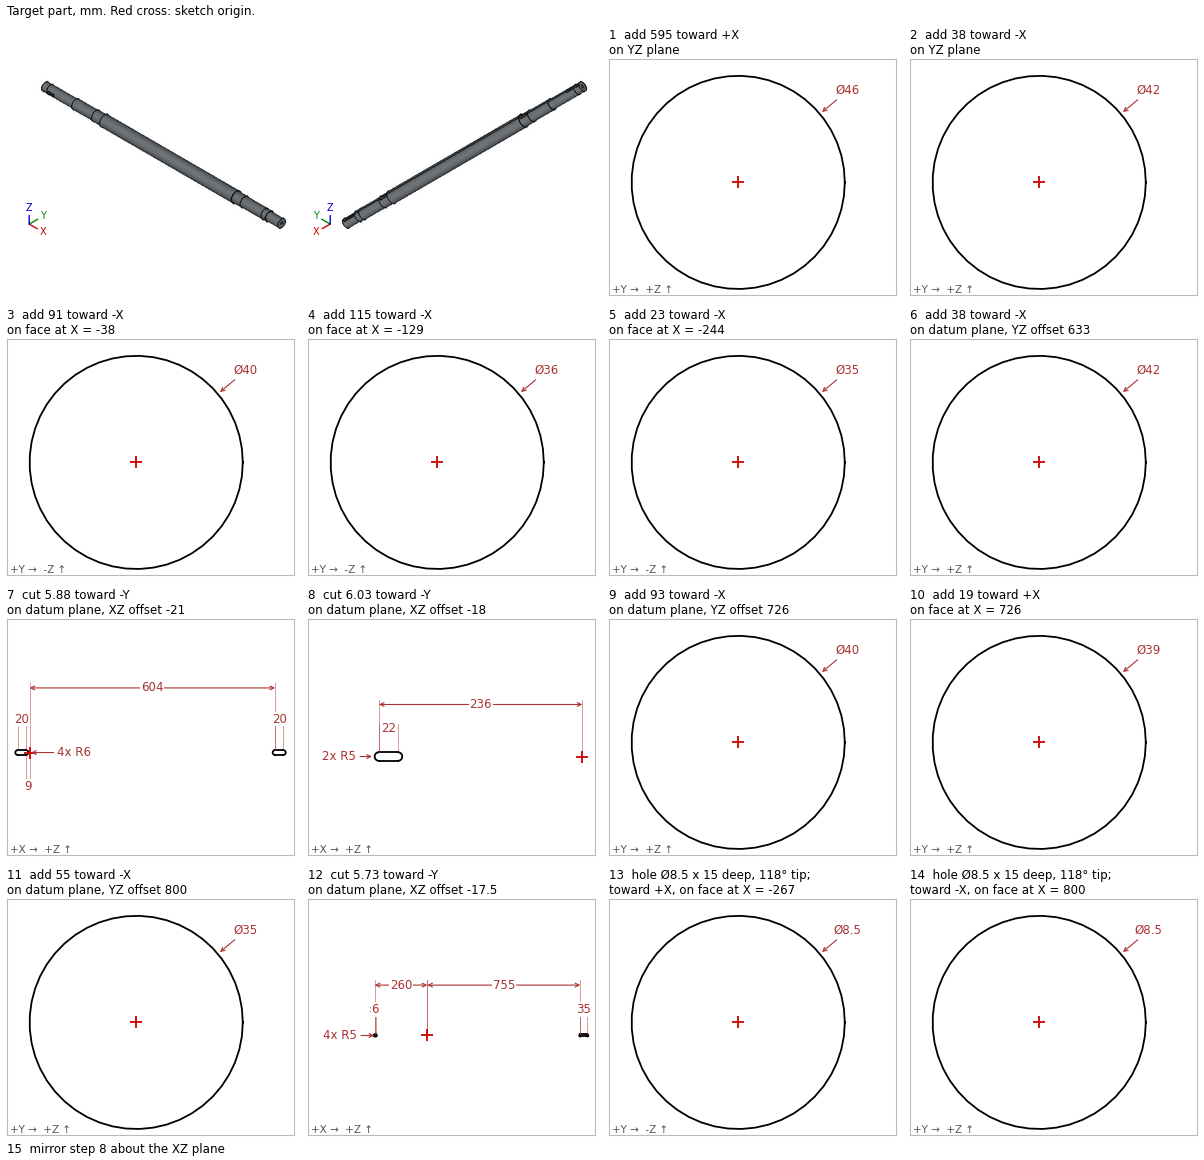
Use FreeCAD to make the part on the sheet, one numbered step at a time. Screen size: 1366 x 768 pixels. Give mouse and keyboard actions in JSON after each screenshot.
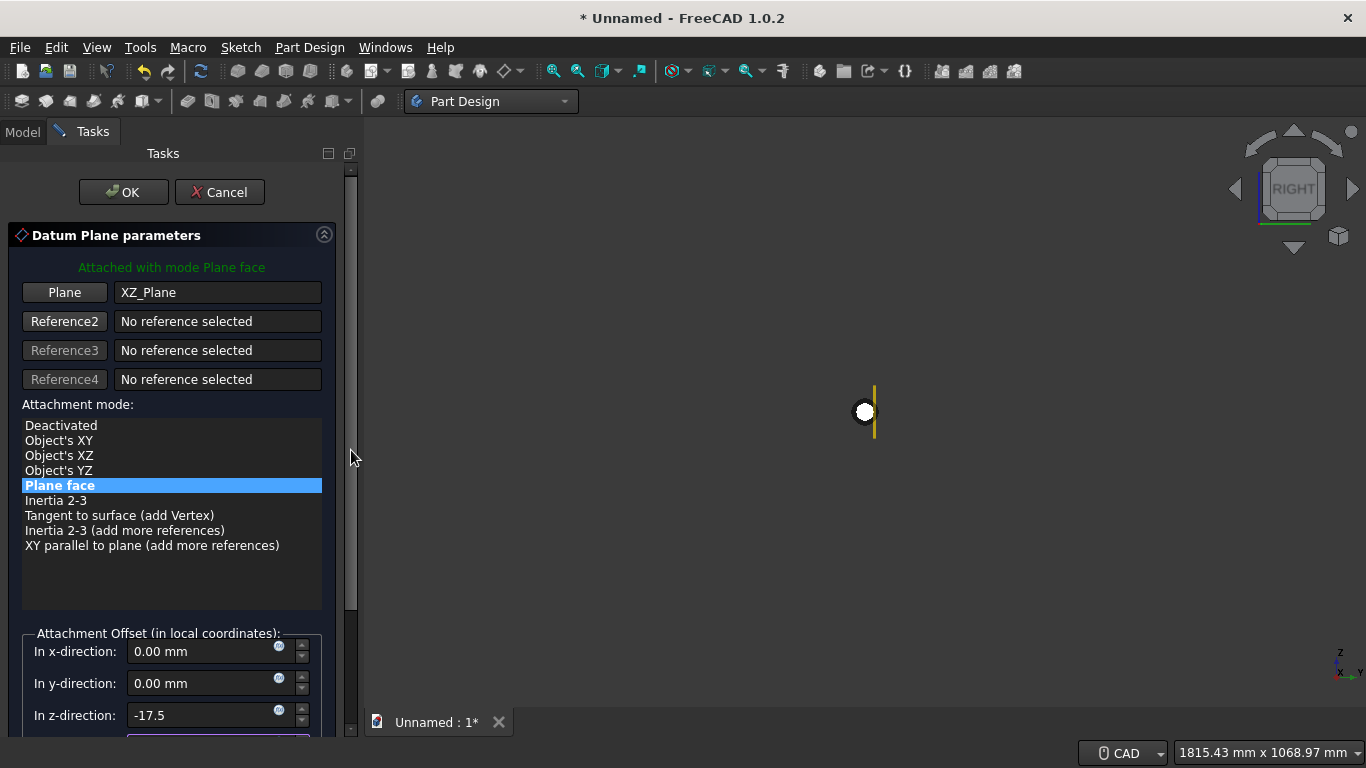
{"action": "left_click", "coordinate": [124, 192]}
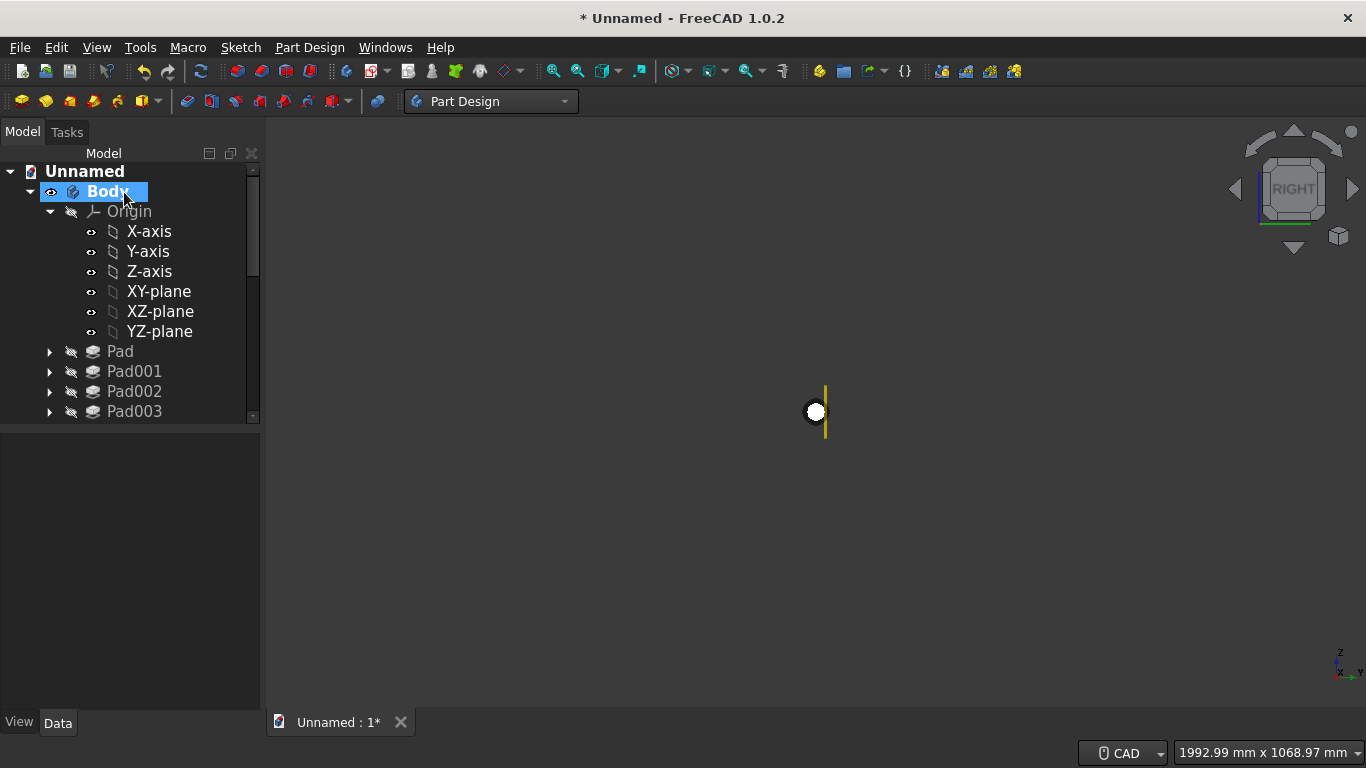
{"action": "scroll", "coordinate": [100, 287], "scroll_direction": "down", "scroll_amount": 3}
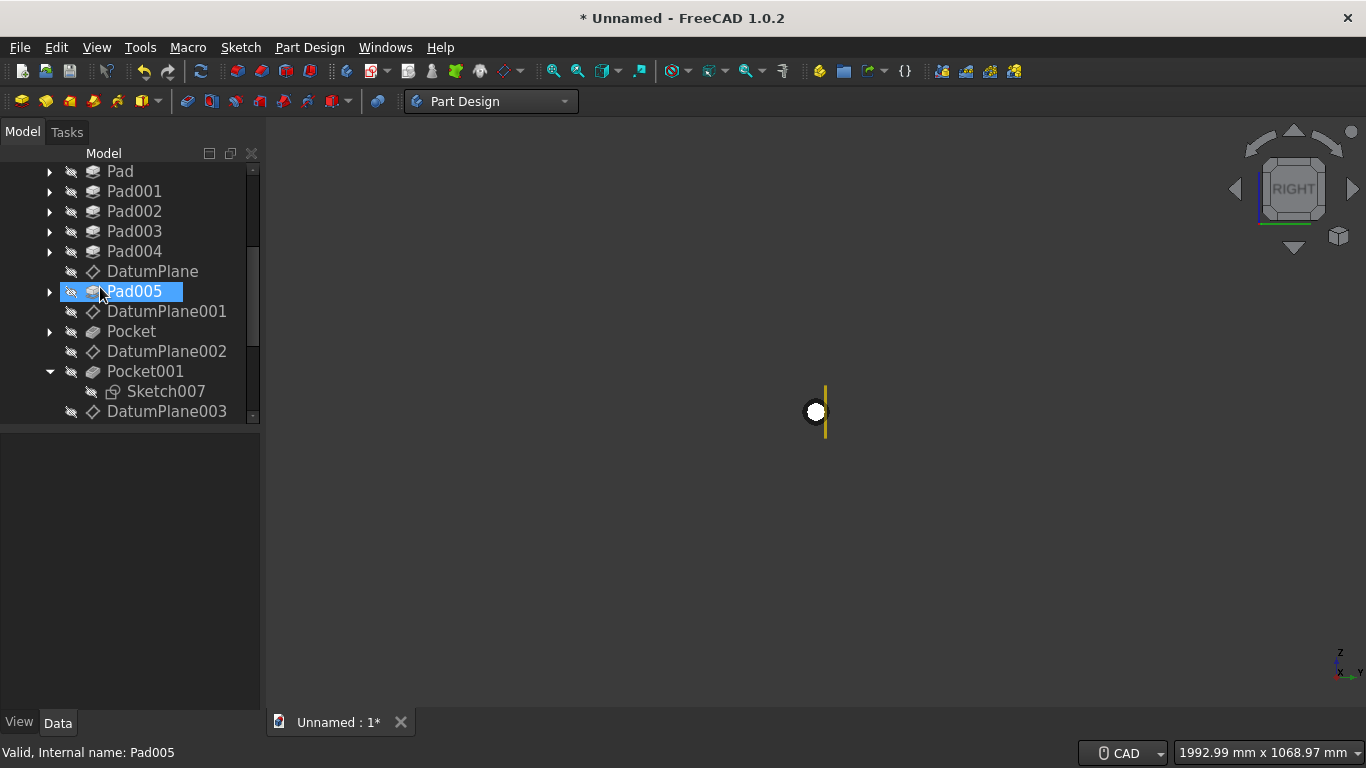
{"action": "scroll", "coordinate": [140, 287], "scroll_direction": "up", "scroll_amount": 15}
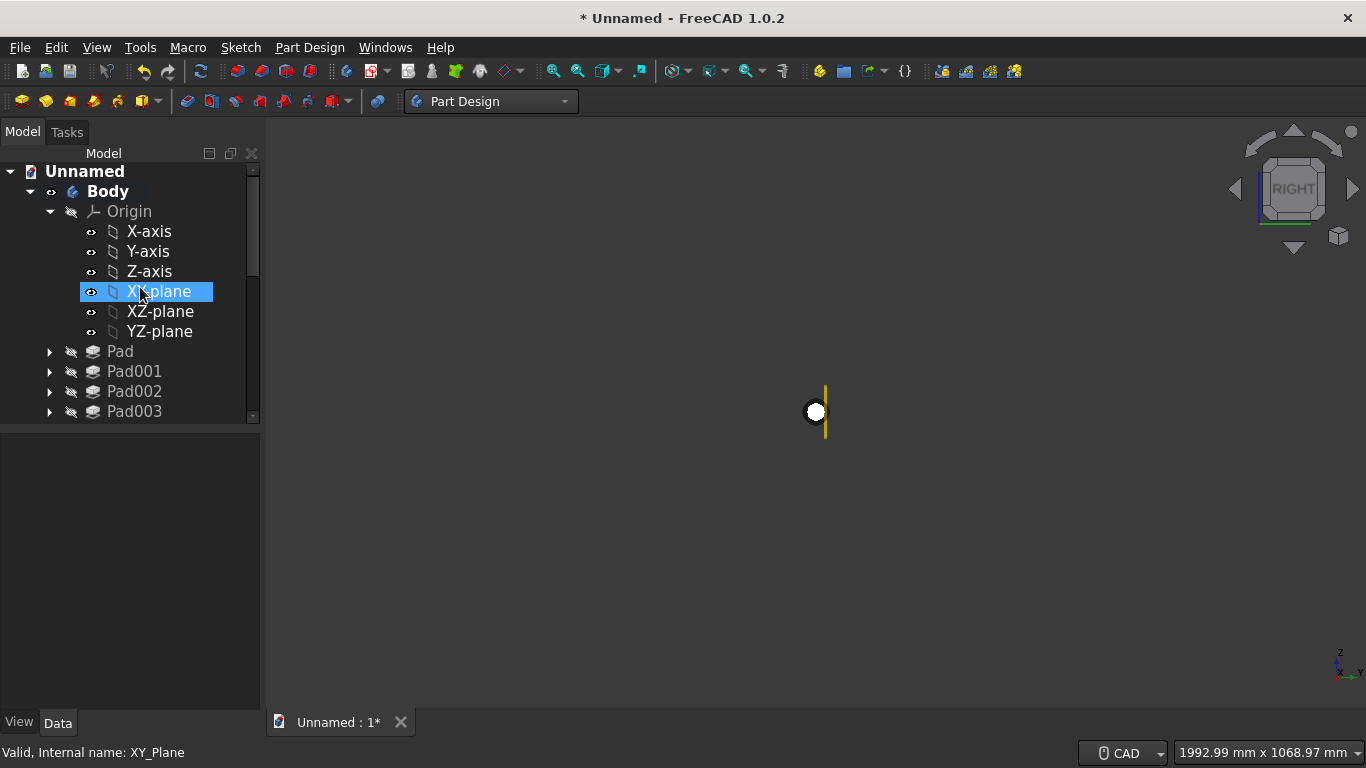
{"action": "scroll", "coordinate": [100, 287], "scroll_direction": "down", "scroll_amount": 6}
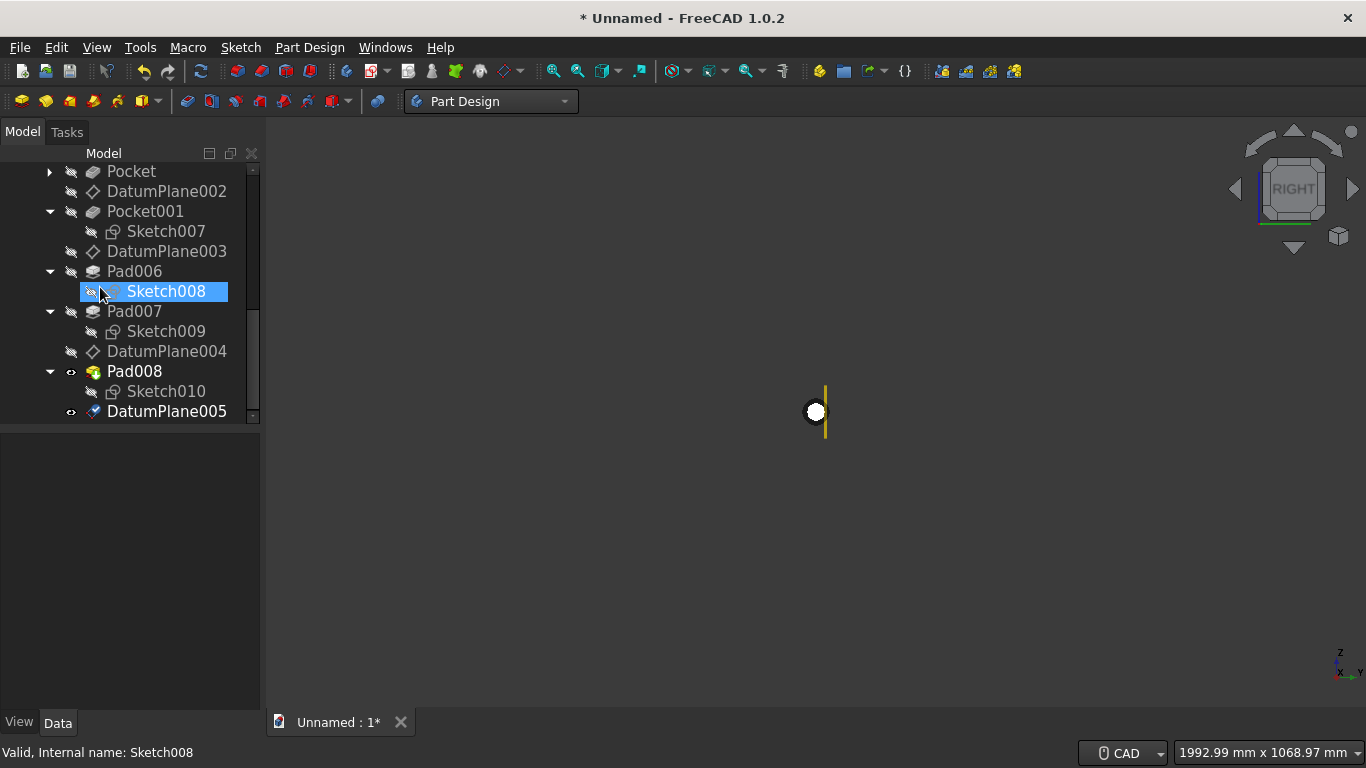
{"action": "left_click", "coordinate": [116, 412]}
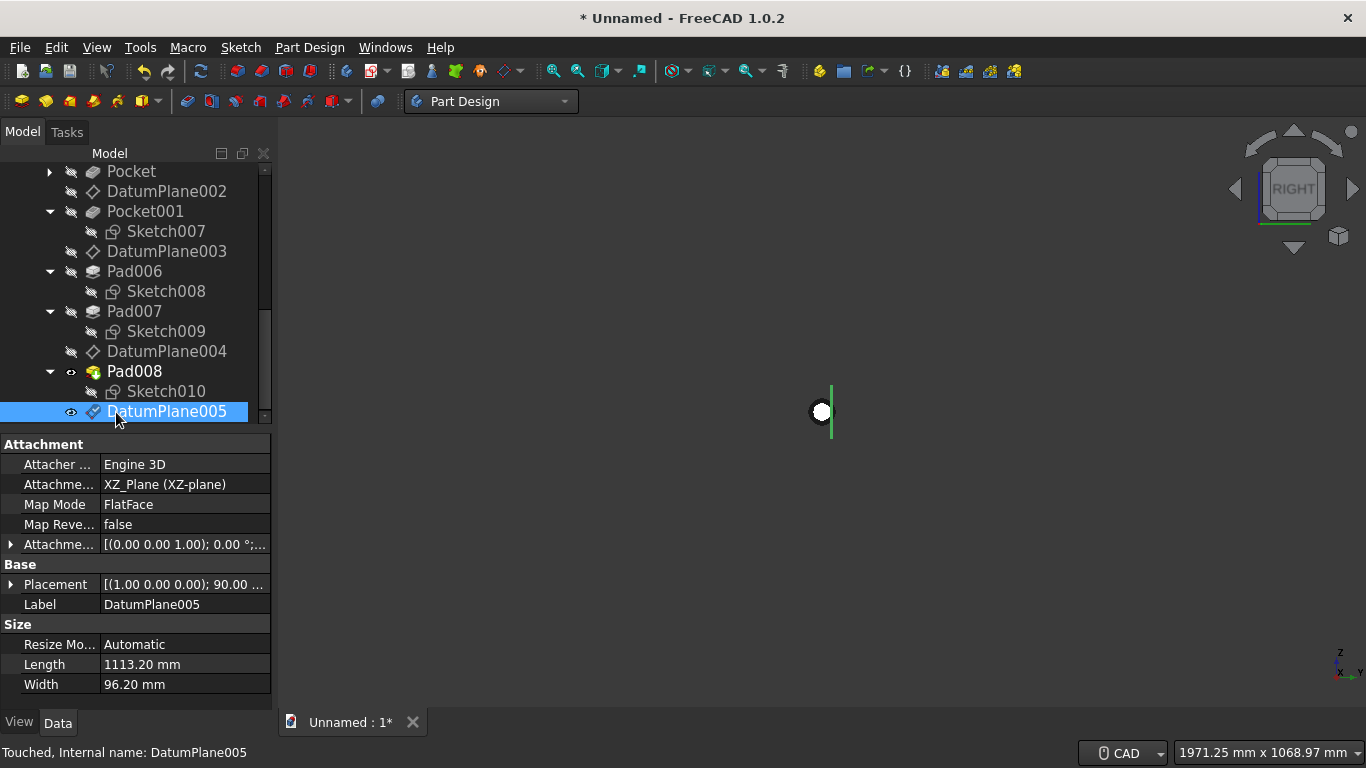
{"action": "left_click", "coordinate": [372, 72]}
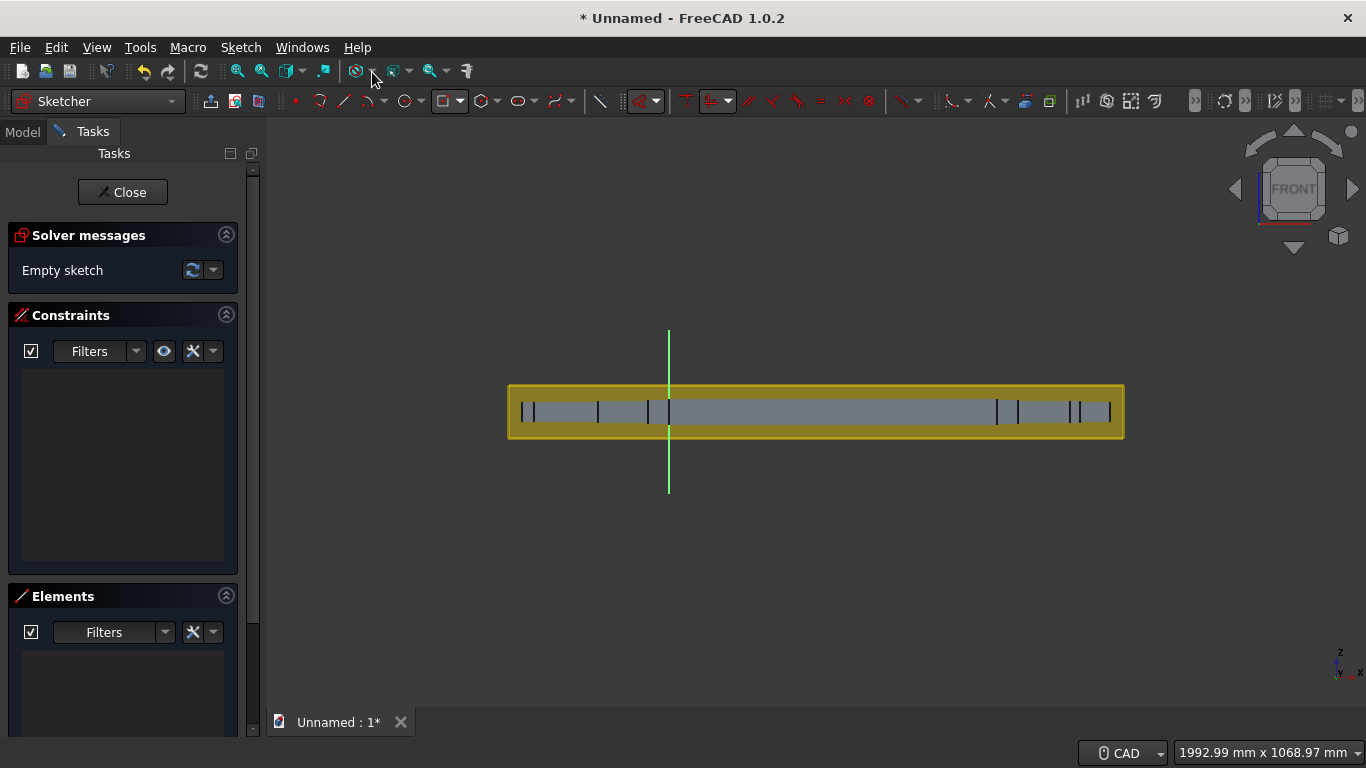
{"action": "key", "text": "q s"}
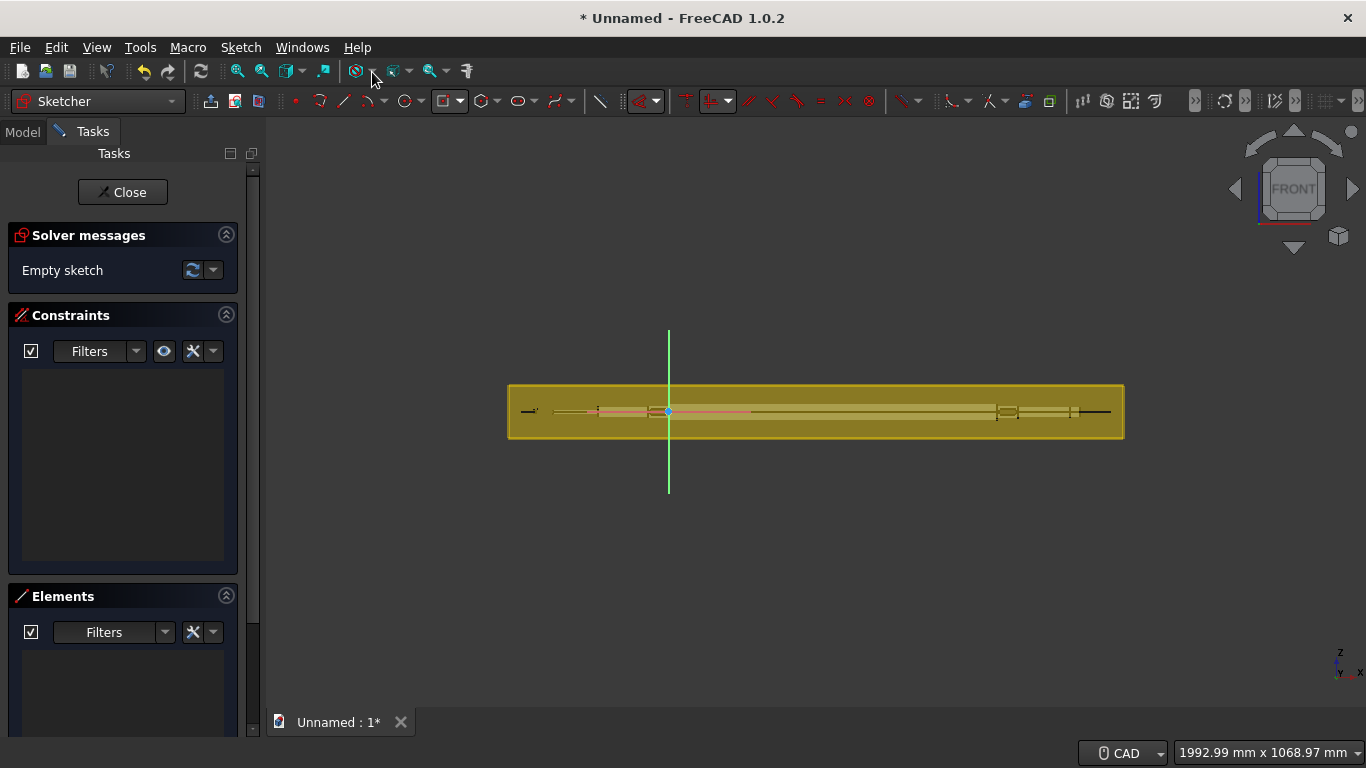
{"action": "key", "text": "g s"}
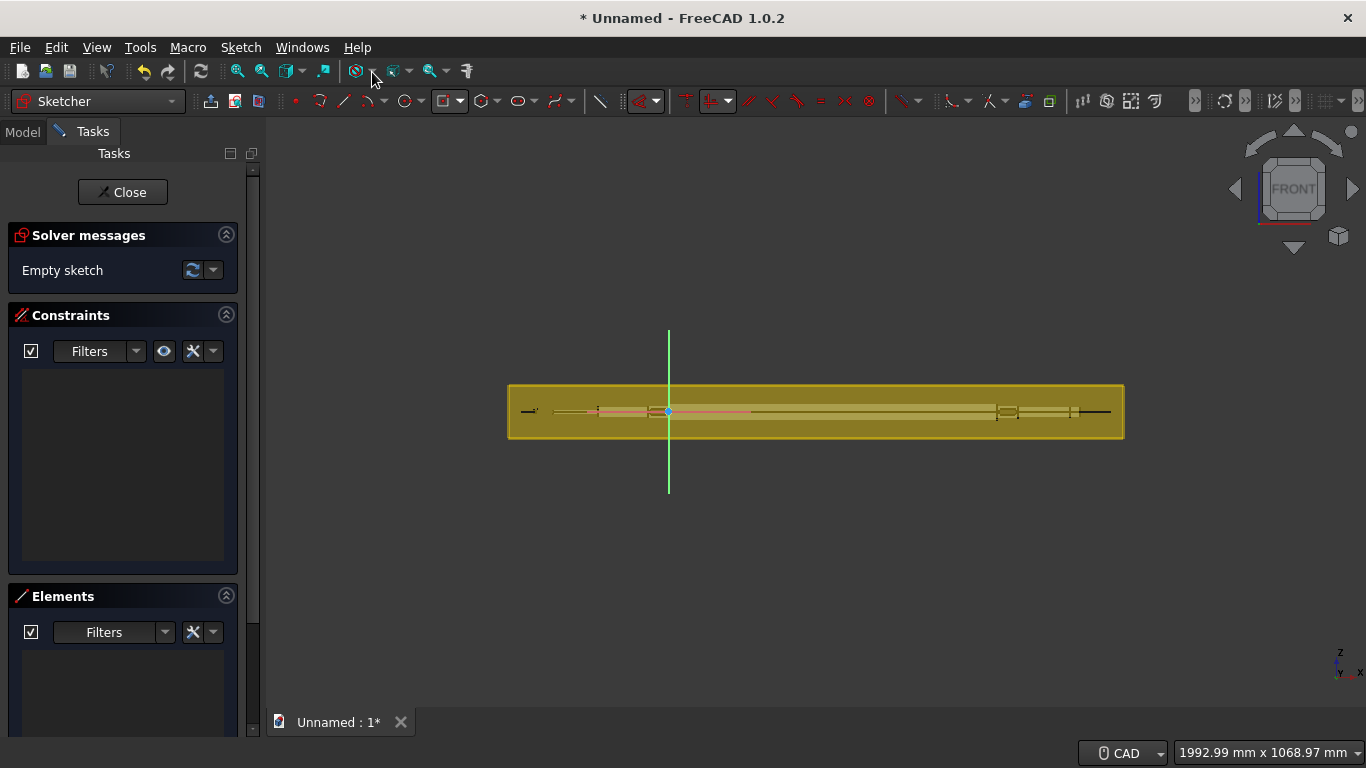
{"action": "scroll", "coordinate": [525, 412], "scroll_direction": "up", "scroll_amount": 11}